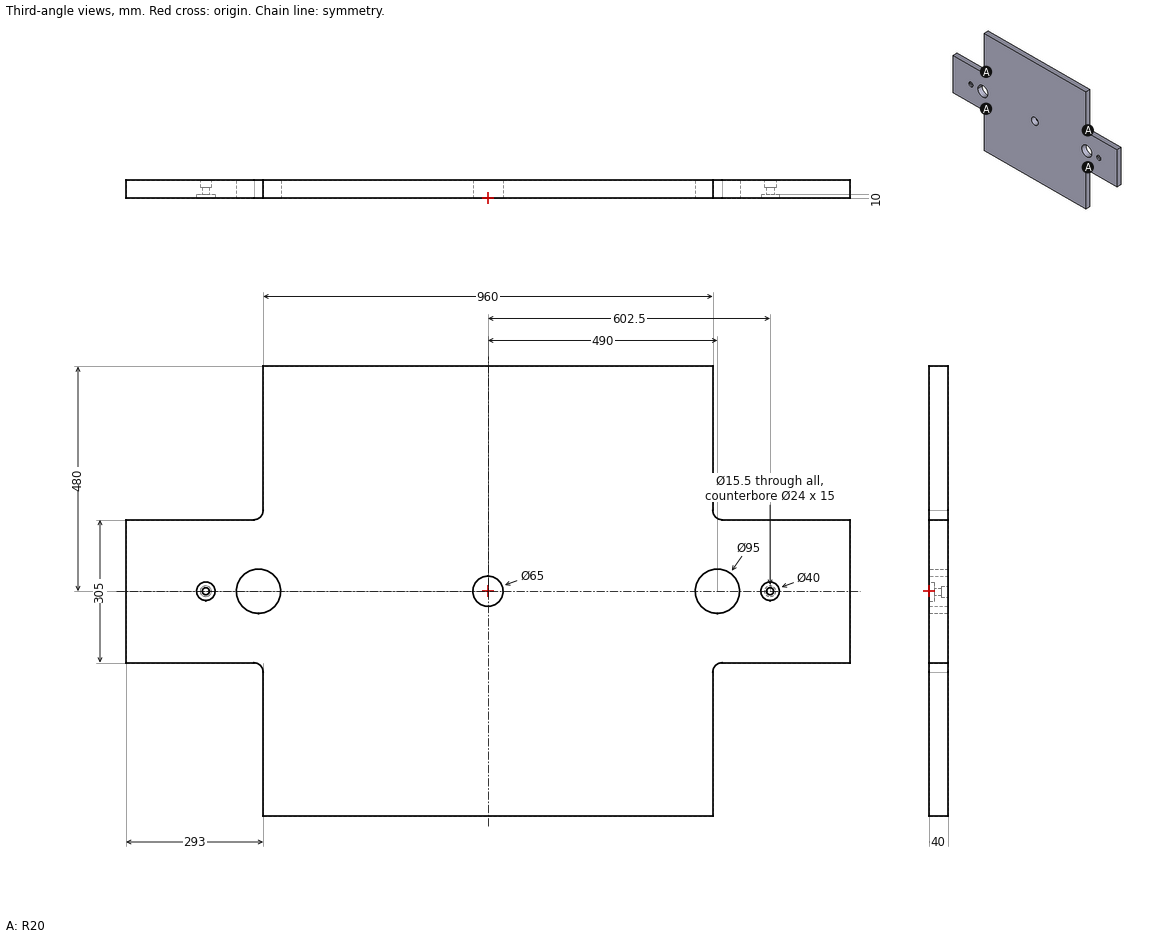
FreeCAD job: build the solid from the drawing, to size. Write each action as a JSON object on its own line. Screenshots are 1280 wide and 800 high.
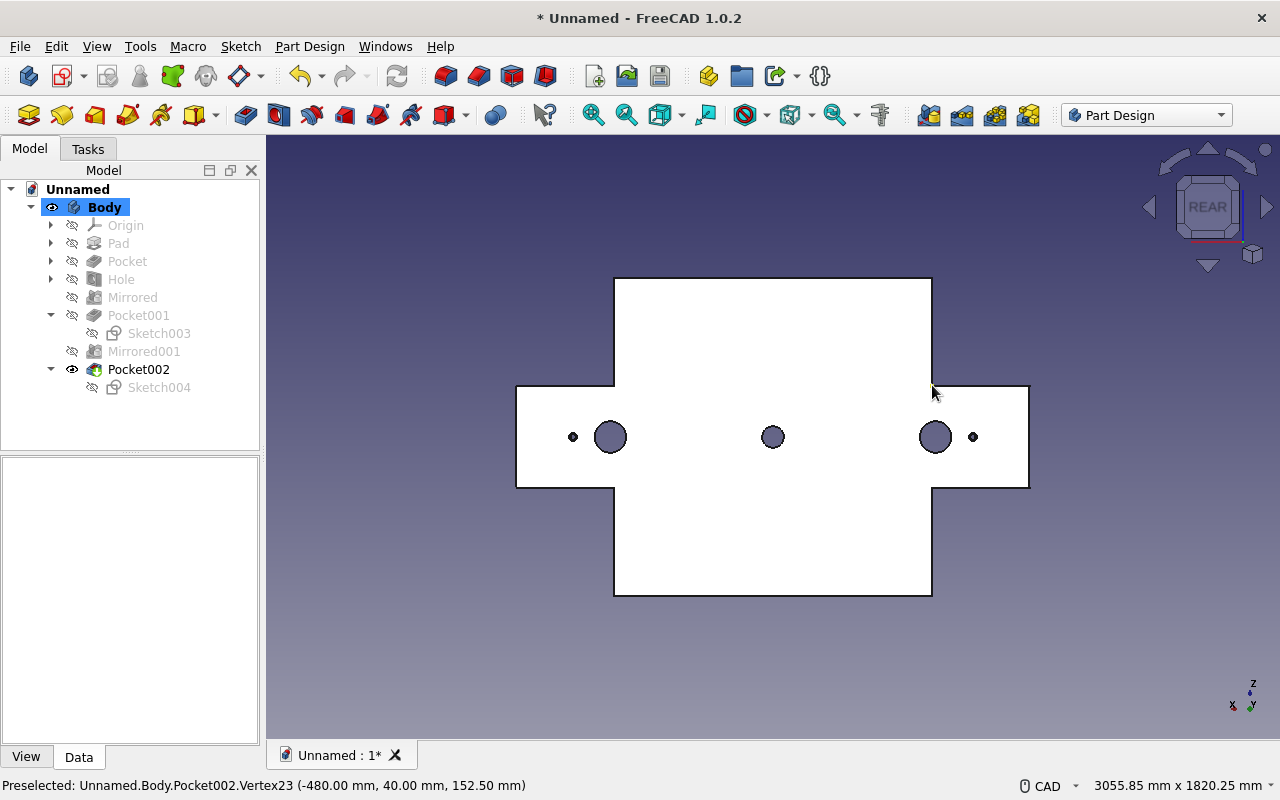
{"action": "key", "text": "6"}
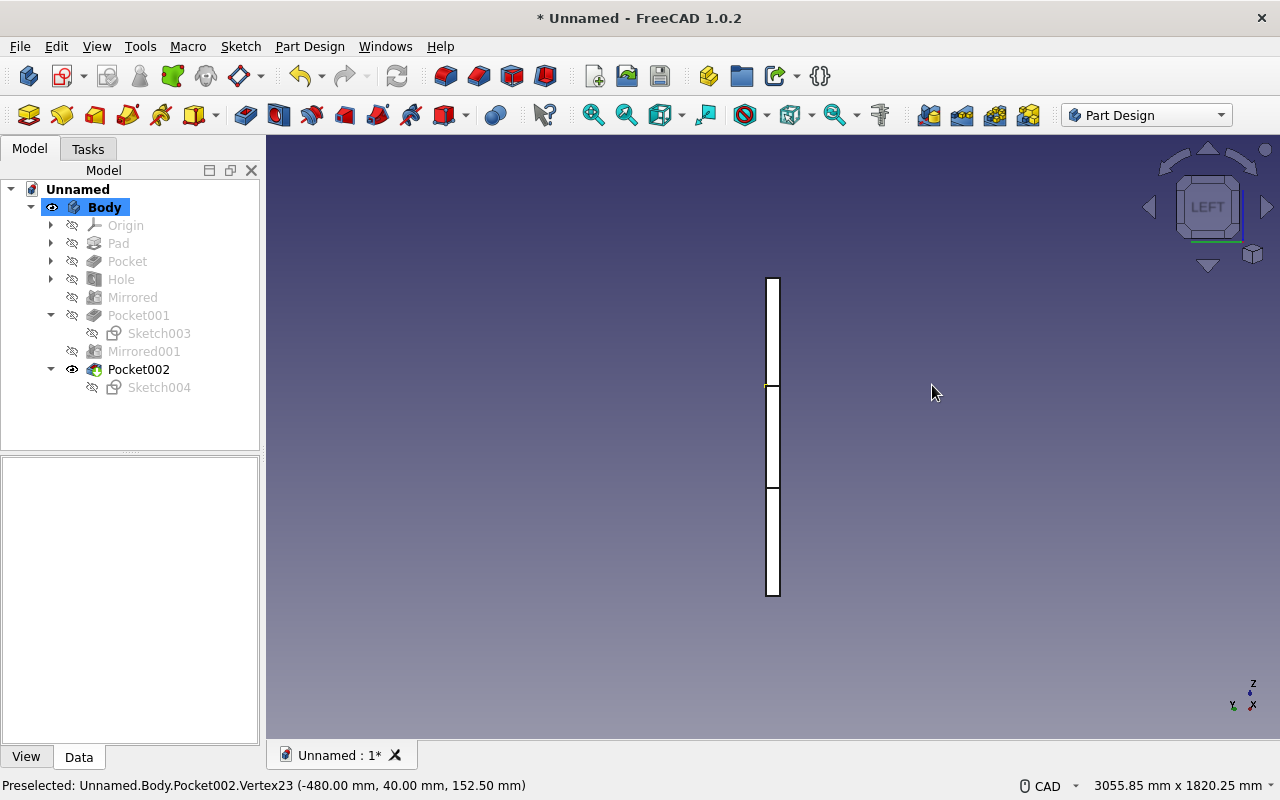
{"action": "scroll", "coordinate": [773, 385], "scroll_direction": "up", "scroll_amount": 6}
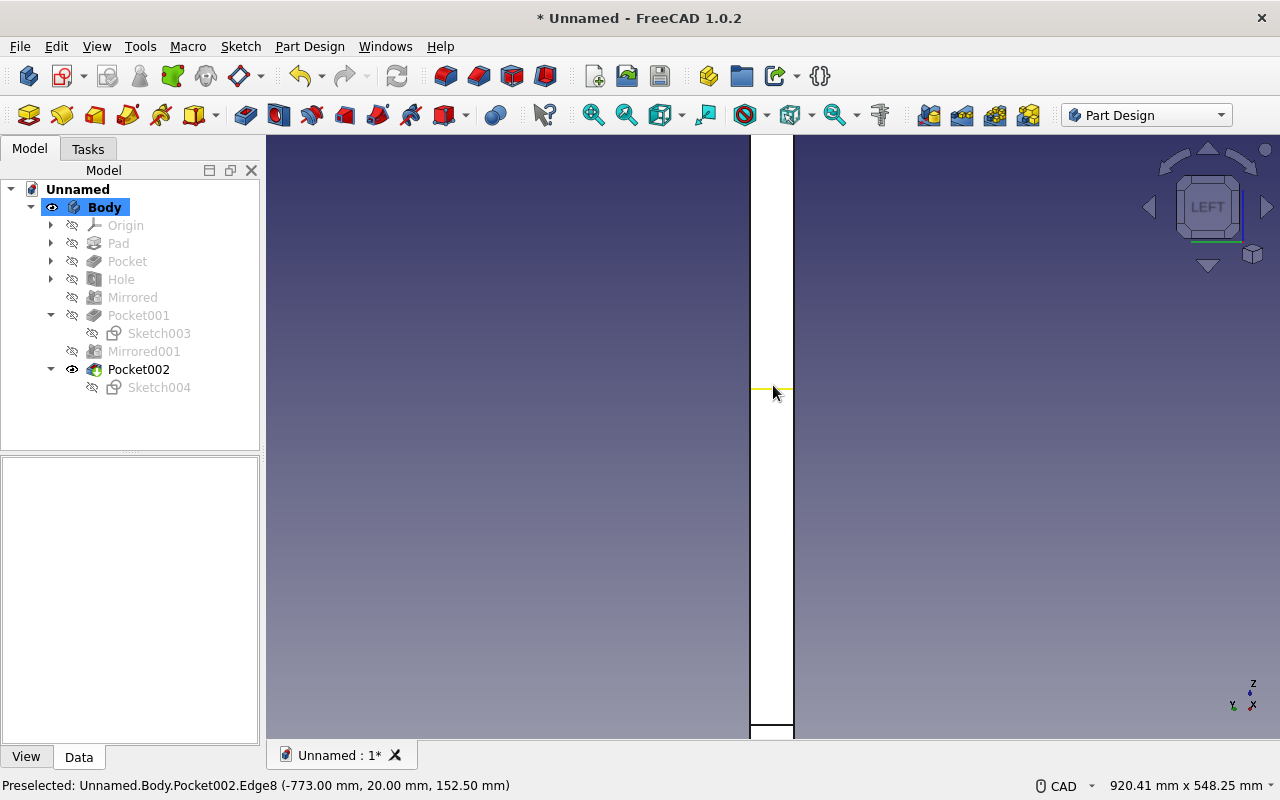
{"action": "key", "text": "v f"}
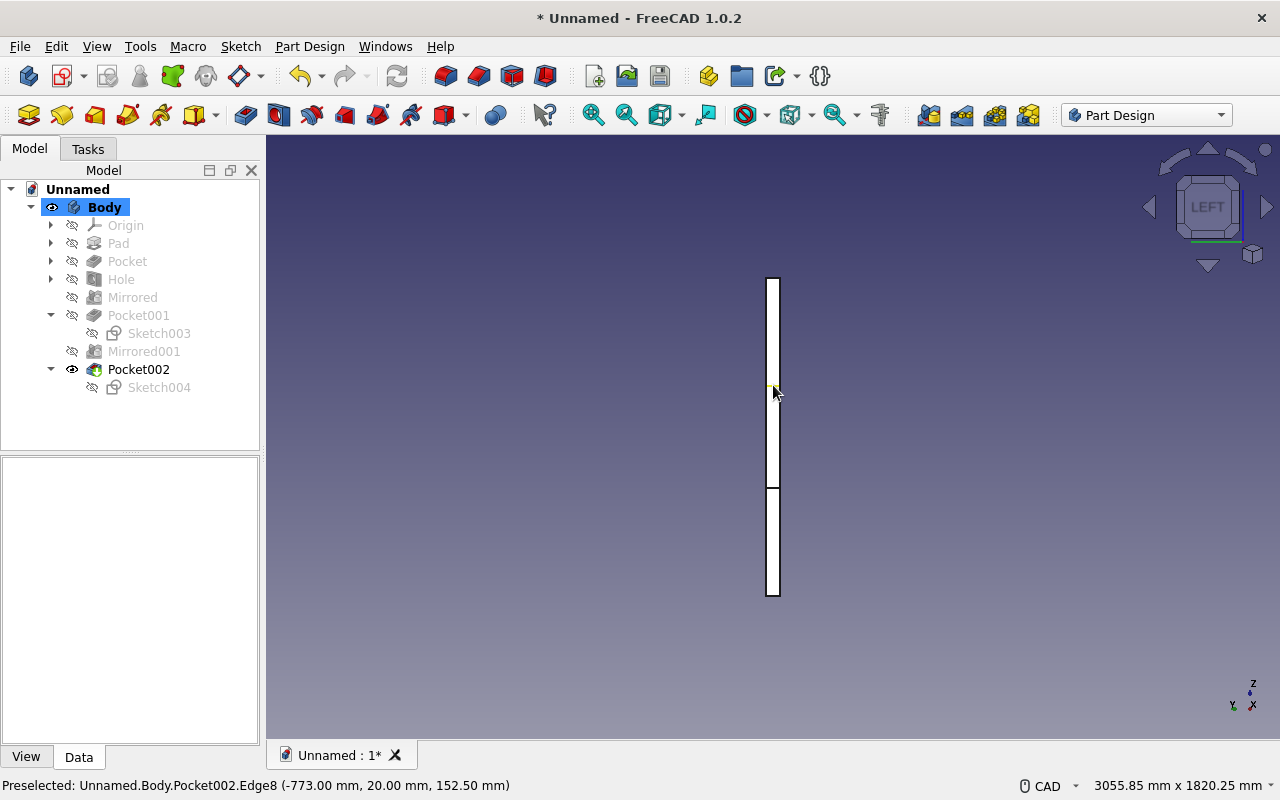
{"action": "key", "text": "v 3"}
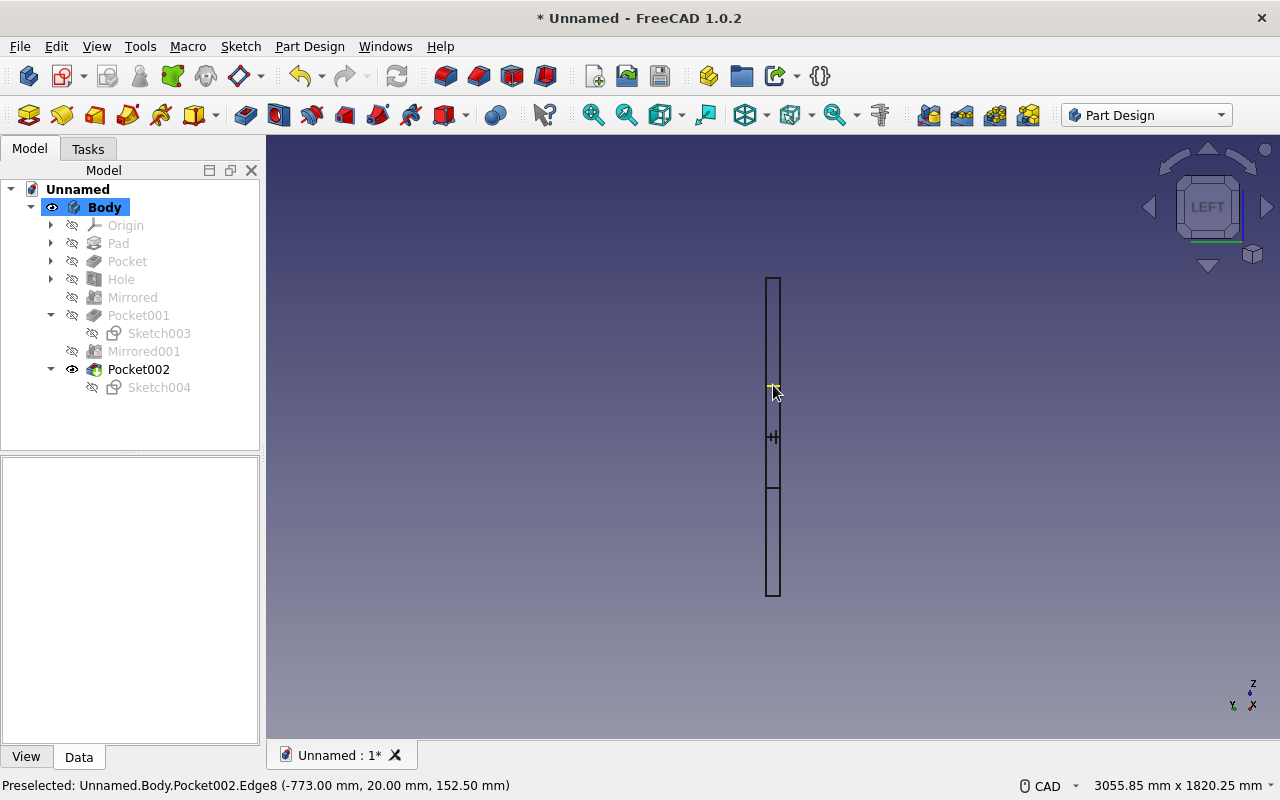
{"action": "key", "text": "0"}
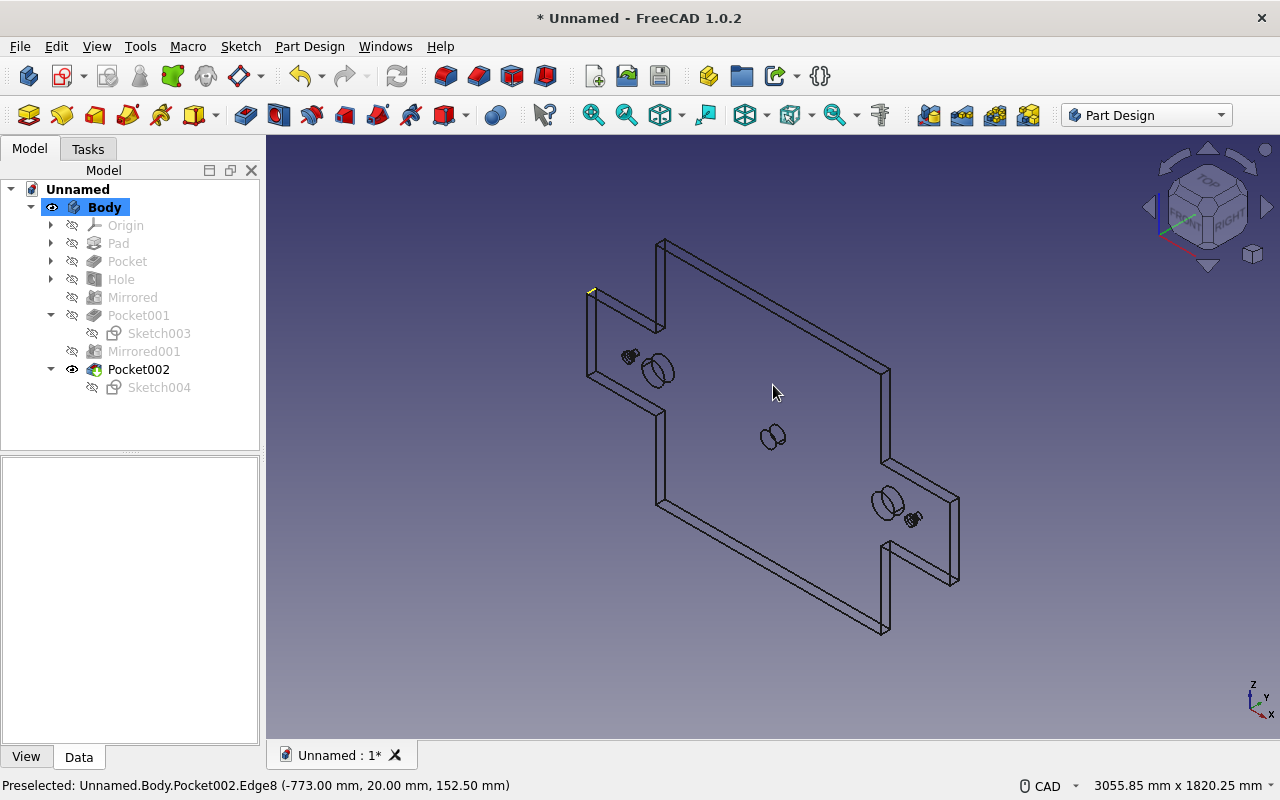
{"action": "left_click", "coordinate": [662, 329]}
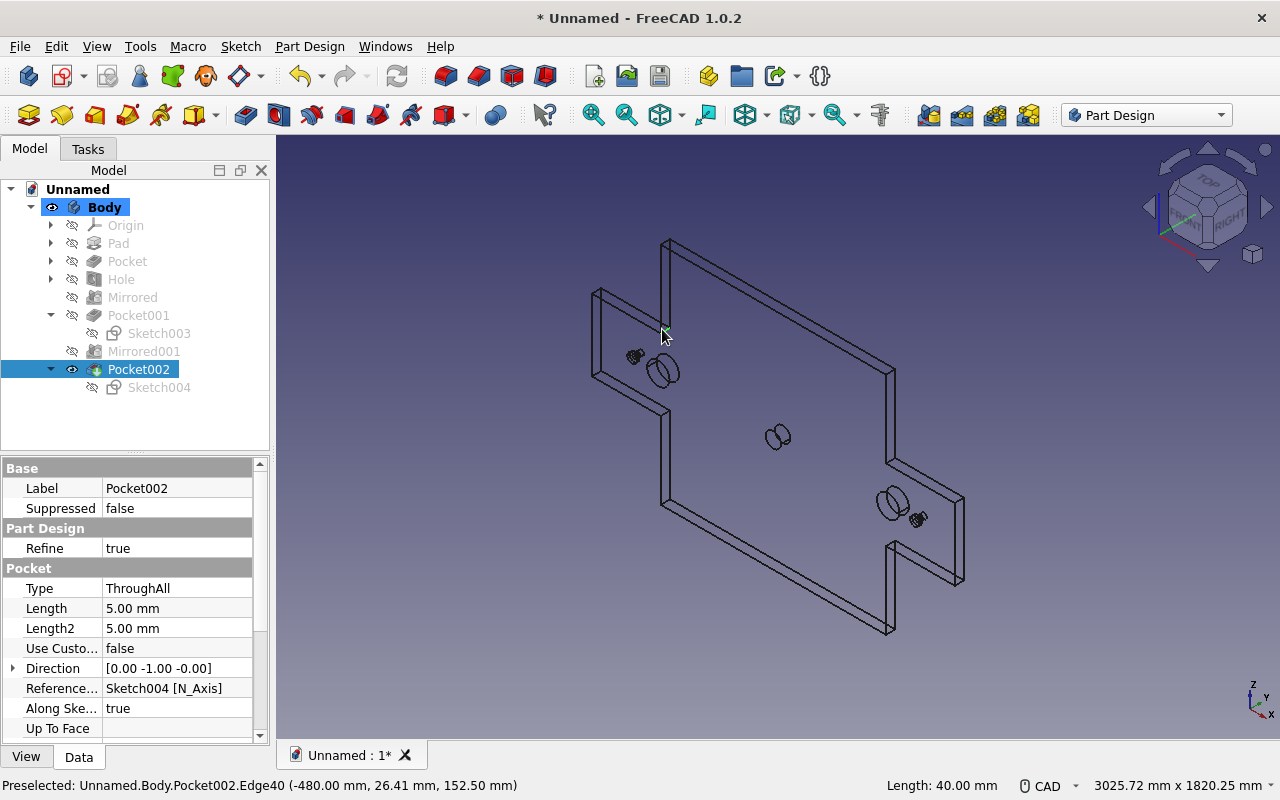
{"action": "left_click", "coordinate": [667, 411], "text": "ctrl"}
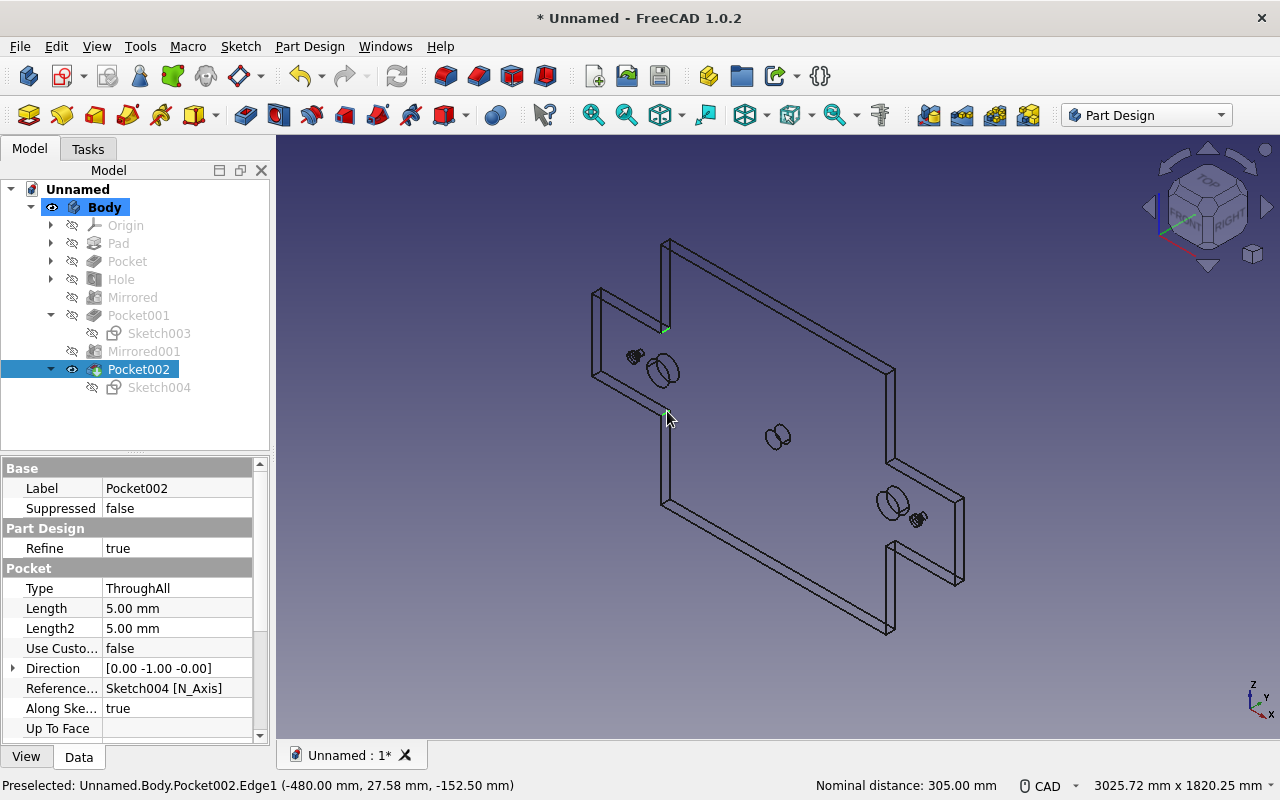
{"action": "left_click", "coordinate": [893, 541], "text": "ctrl"}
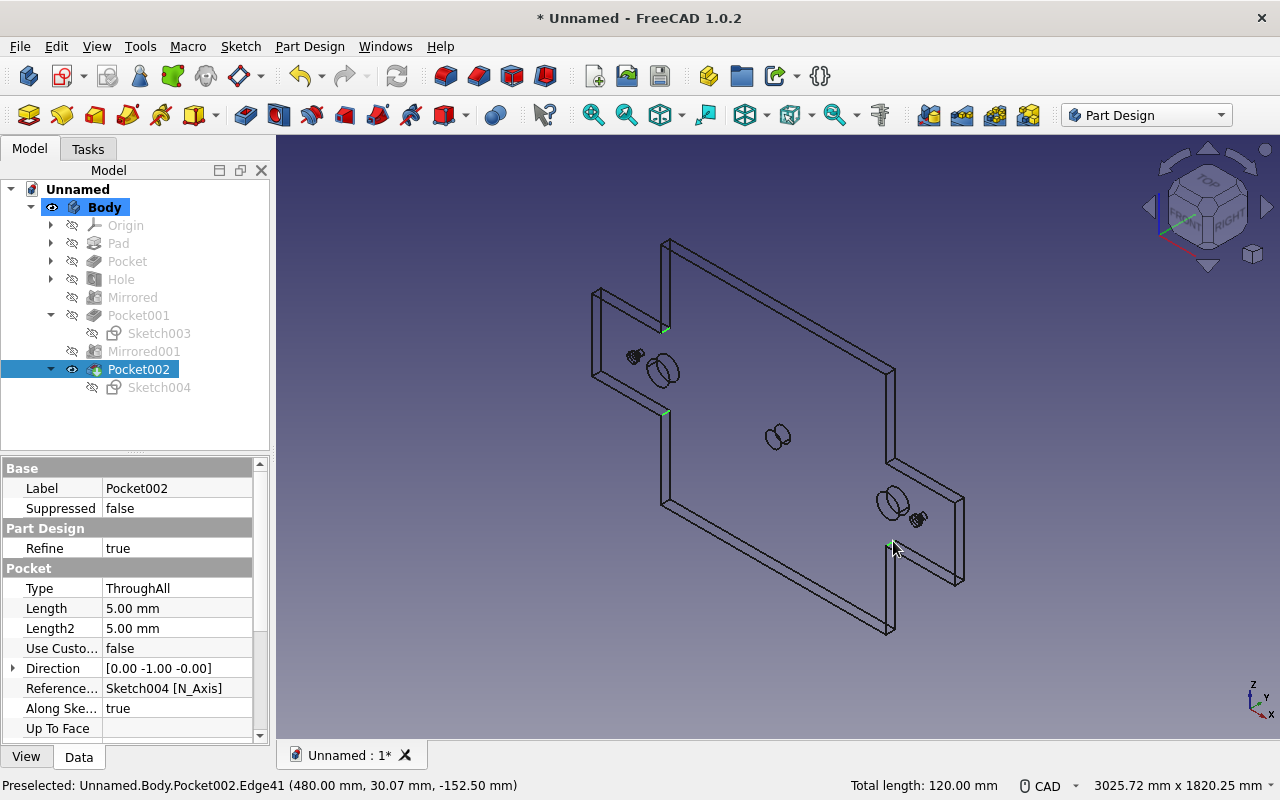
{"action": "left_click", "coordinate": [893, 459], "text": "ctrl"}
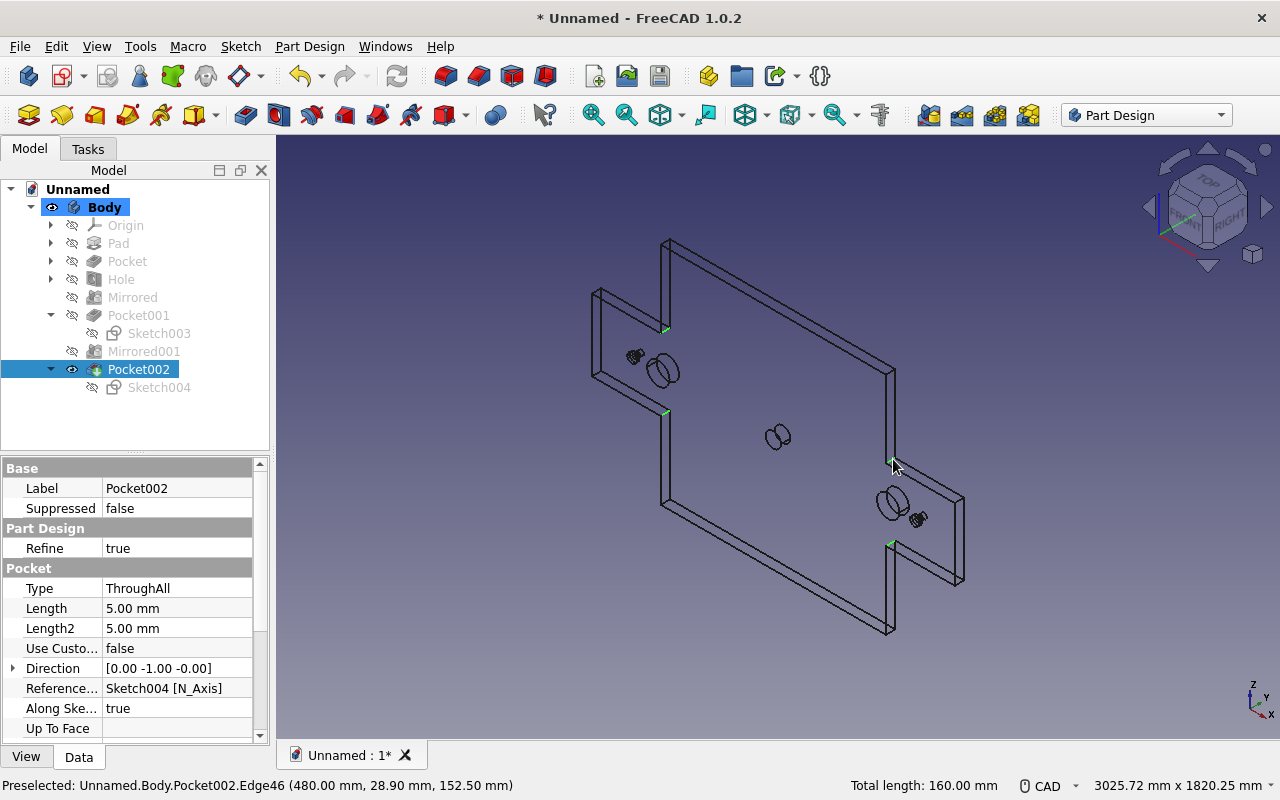
{"action": "key", "text": "v 1"}